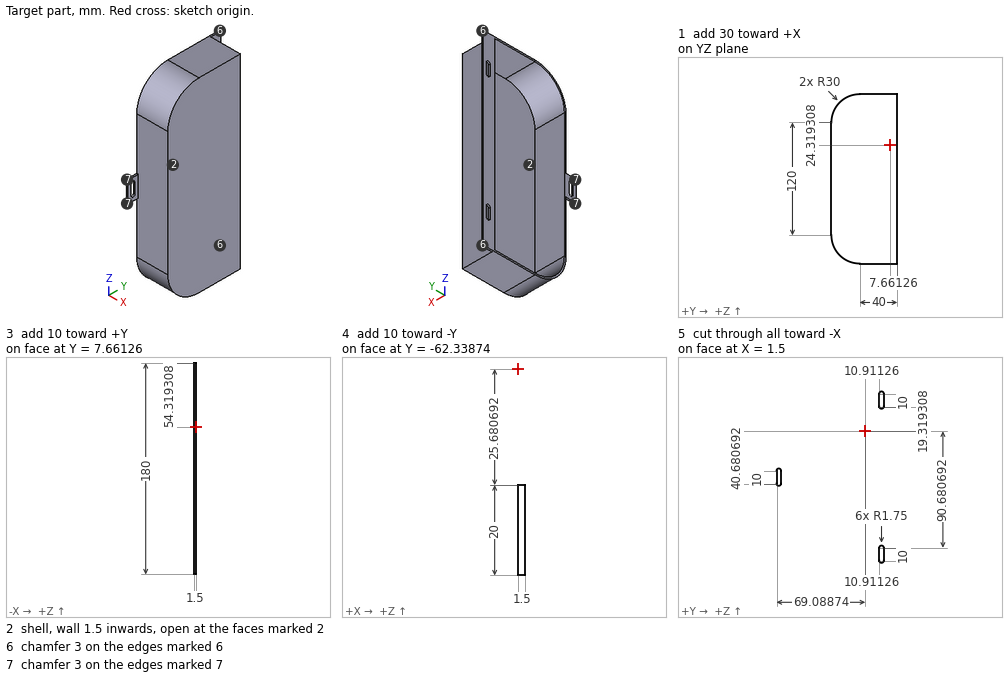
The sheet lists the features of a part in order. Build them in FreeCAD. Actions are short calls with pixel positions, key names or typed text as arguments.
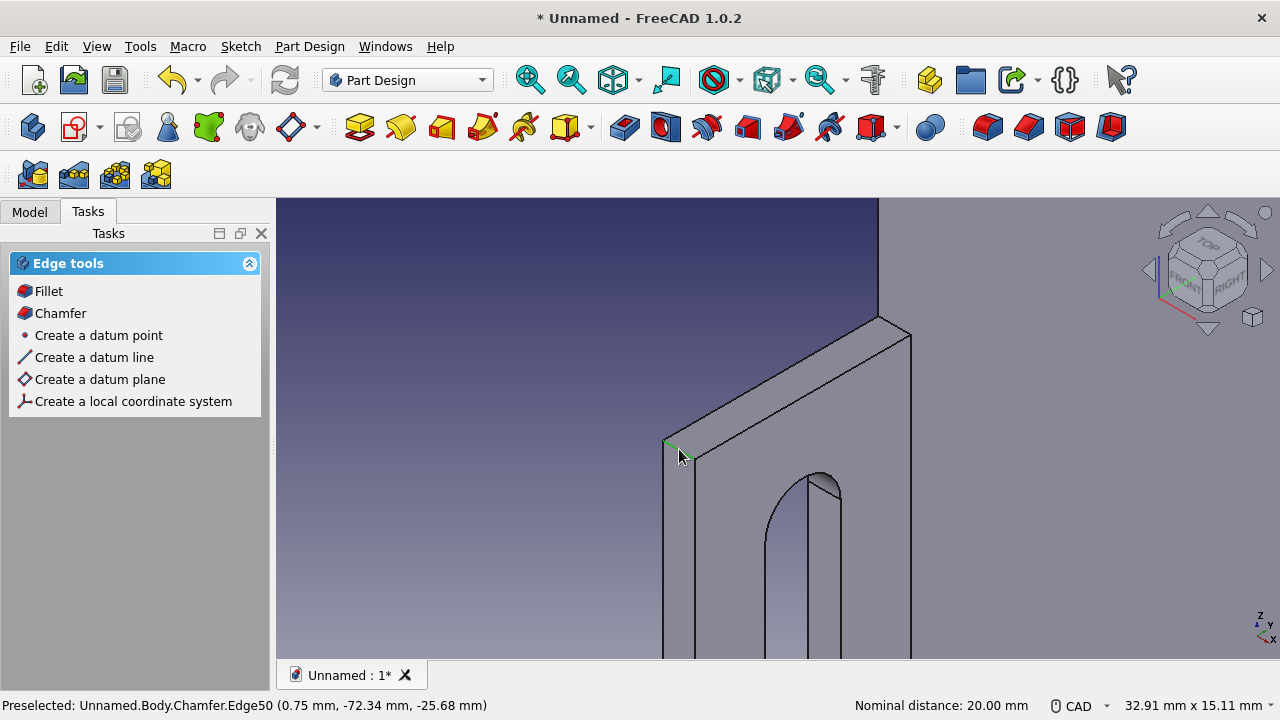
click(1029, 128)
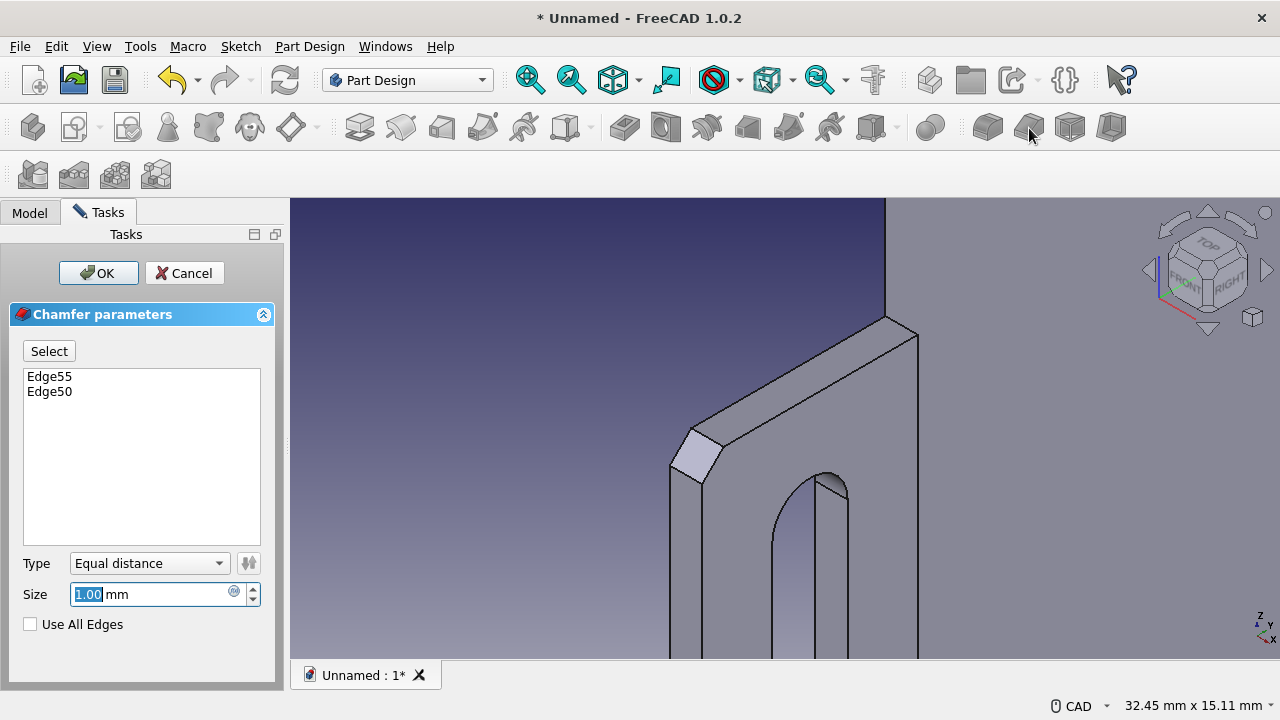
text(3)
key(Tab)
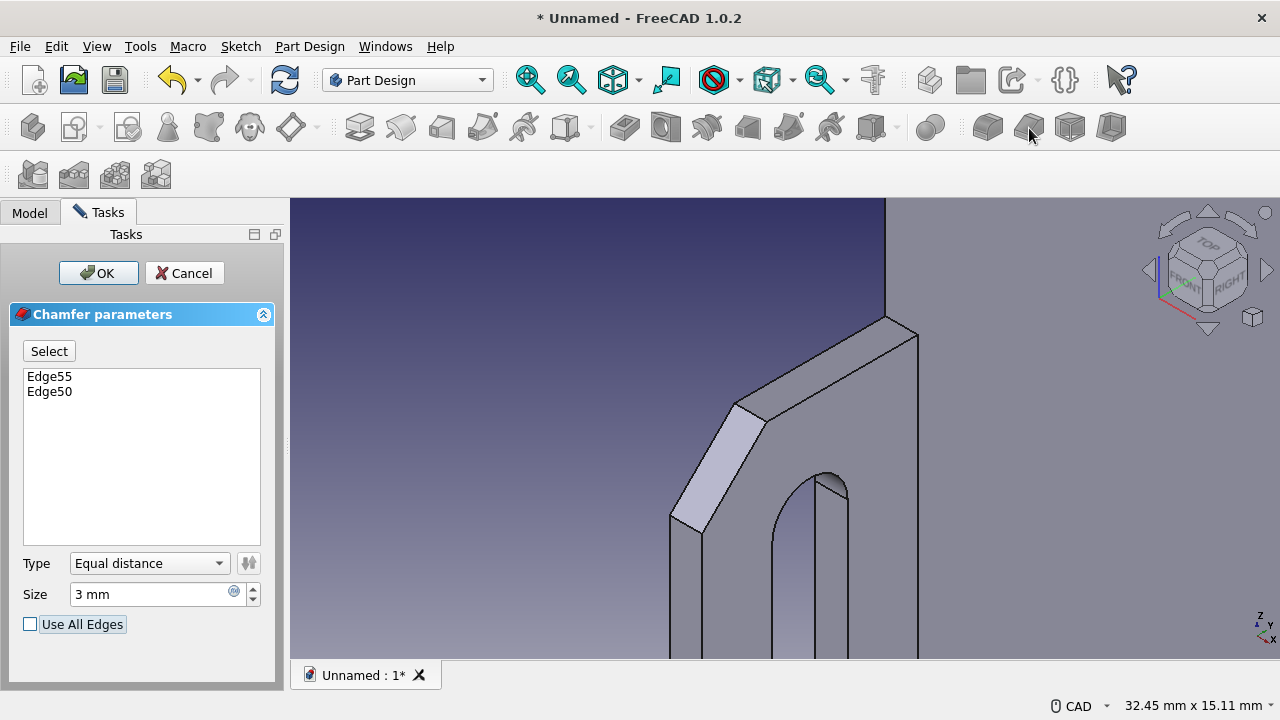
click(99, 273)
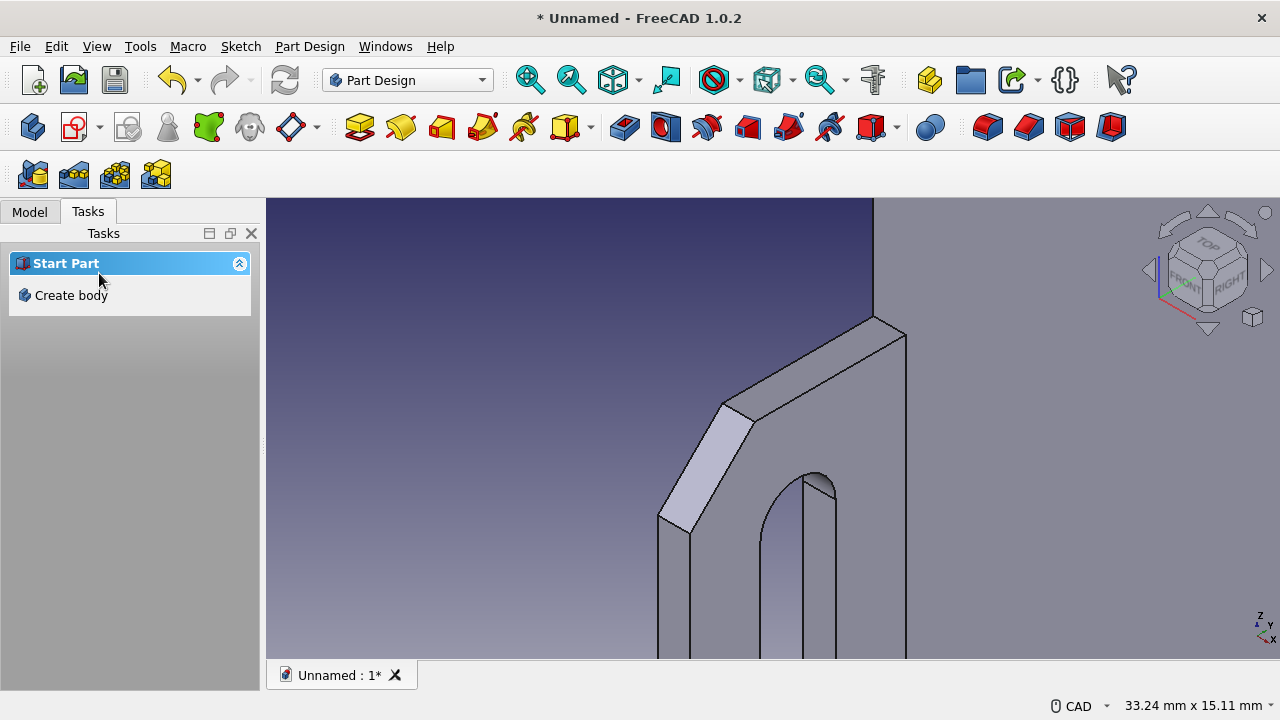
click(531, 80)